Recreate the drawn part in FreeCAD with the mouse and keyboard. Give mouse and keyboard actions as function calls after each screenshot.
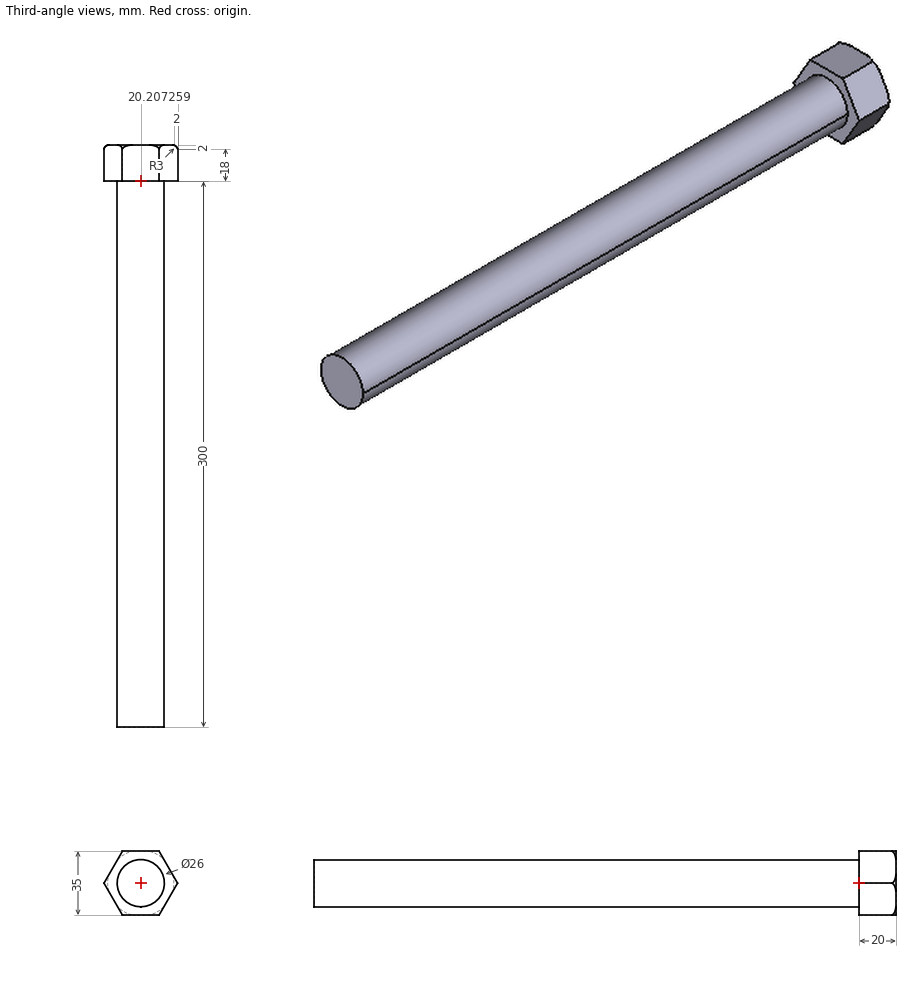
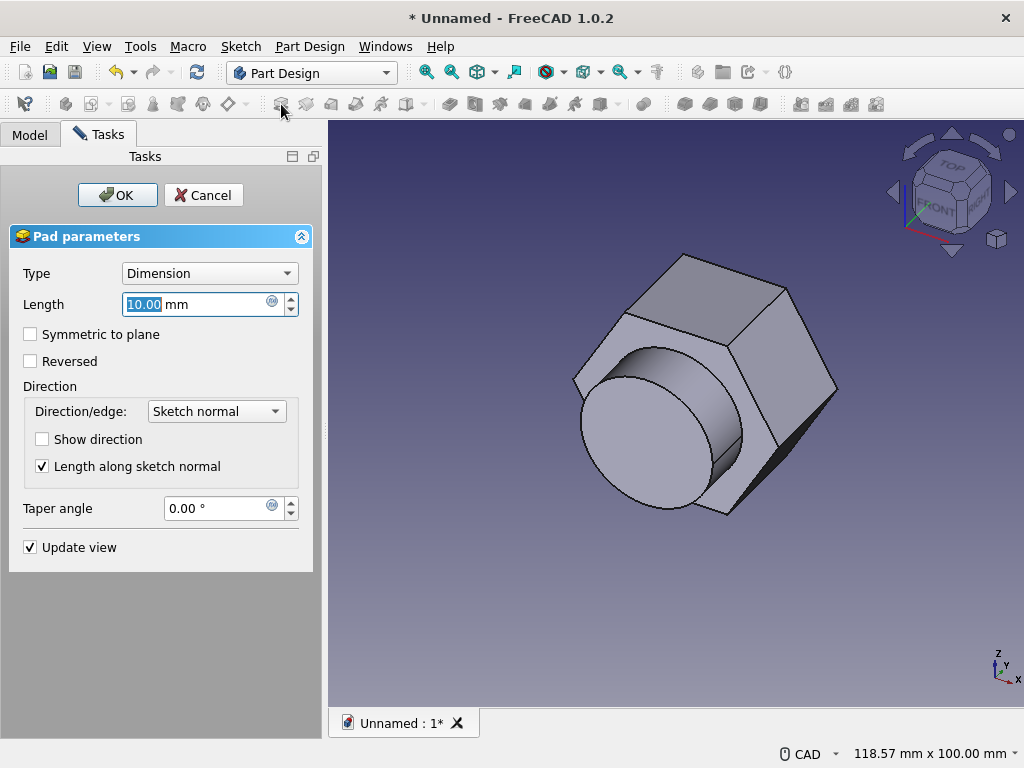
text(300)
key(Tab)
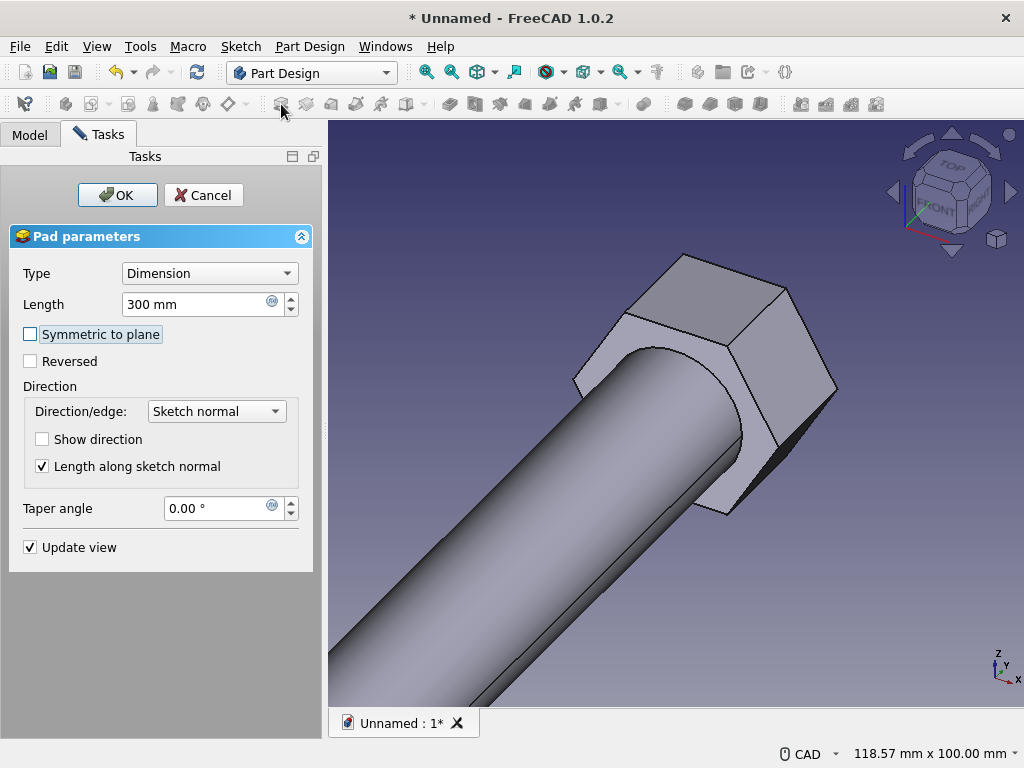
click(118, 195)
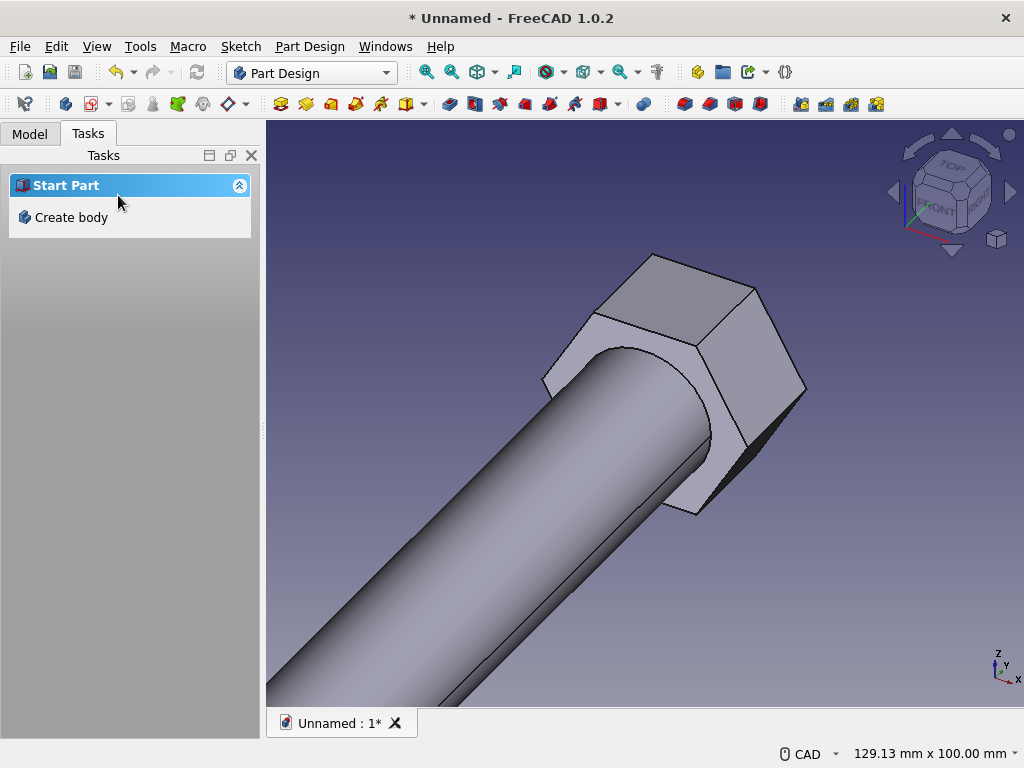
click(427, 72)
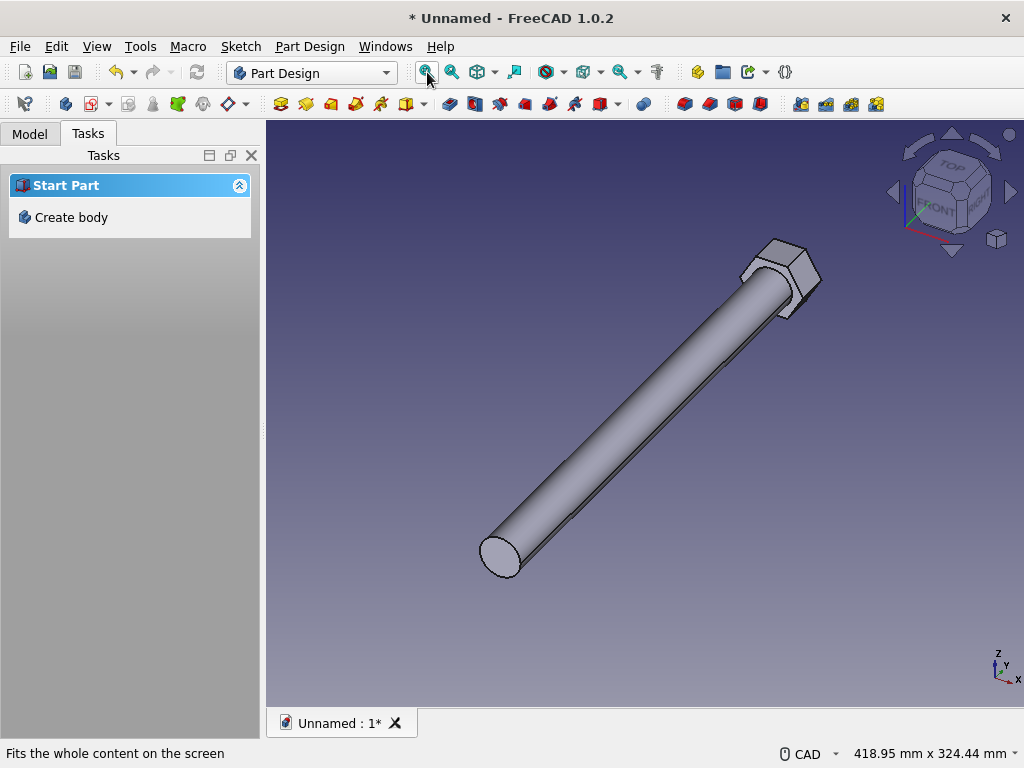
click(90, 104)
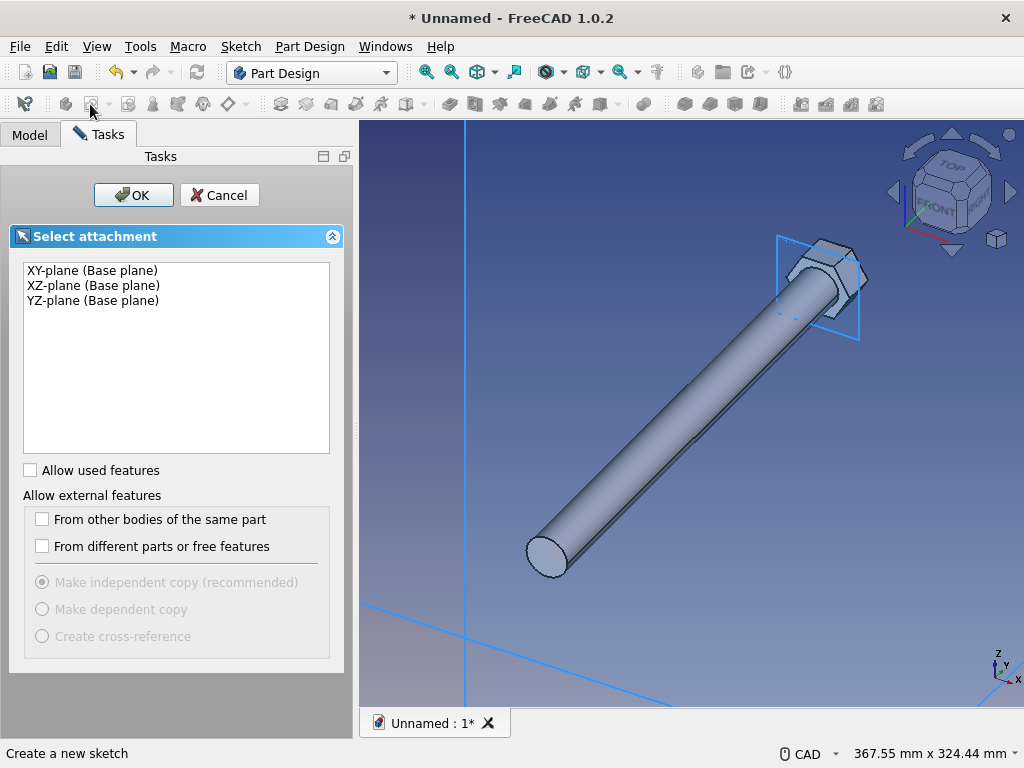
click(84, 270)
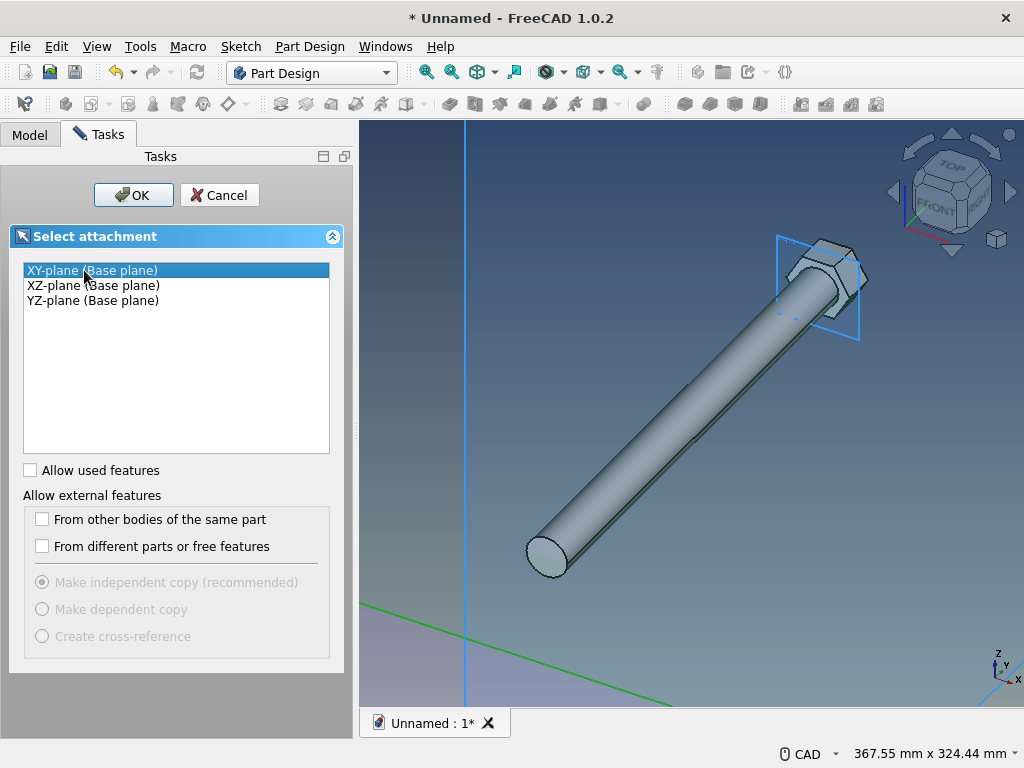
click(134, 195)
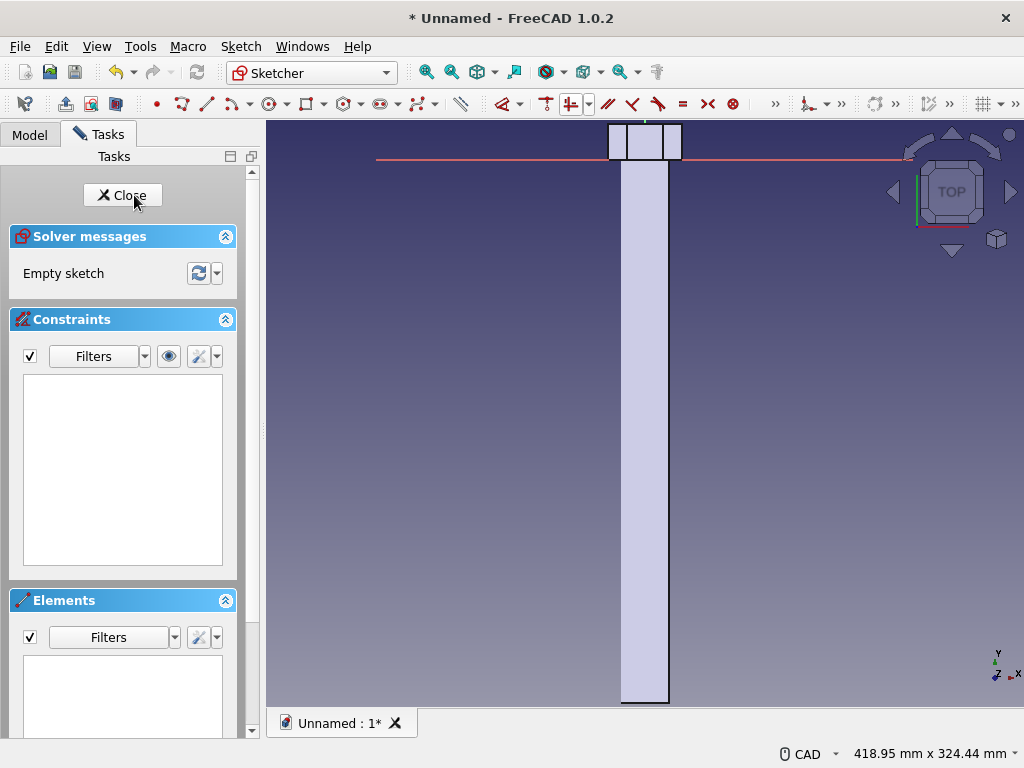
click(116, 104)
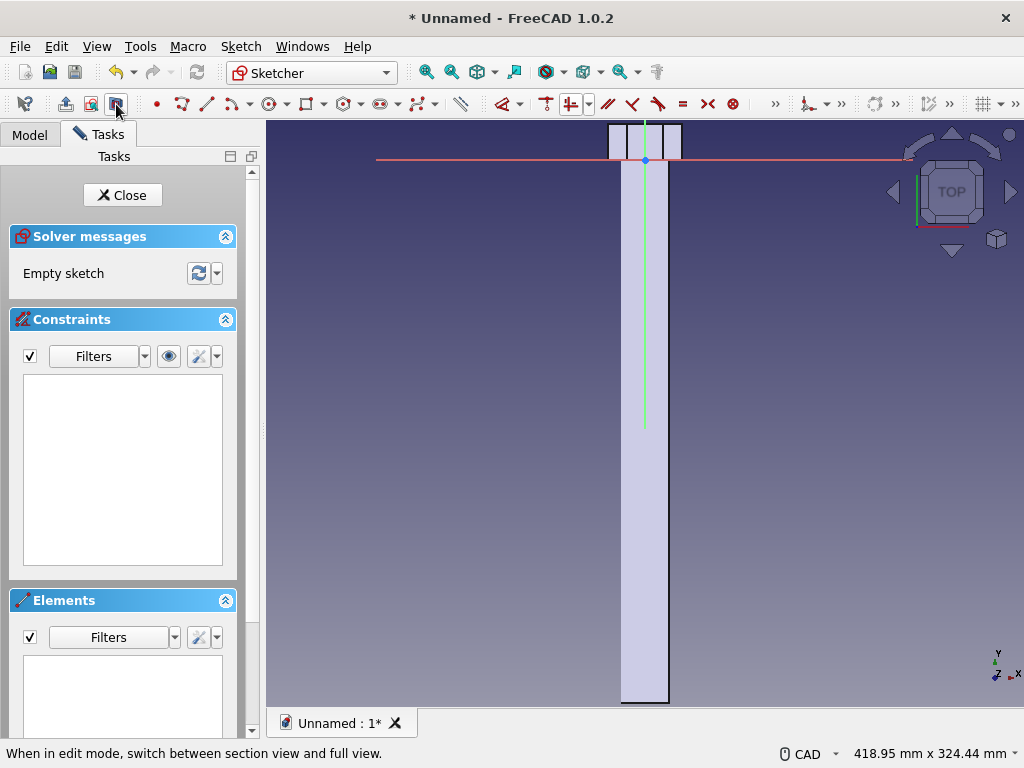
scroll(576, 414, down, 5)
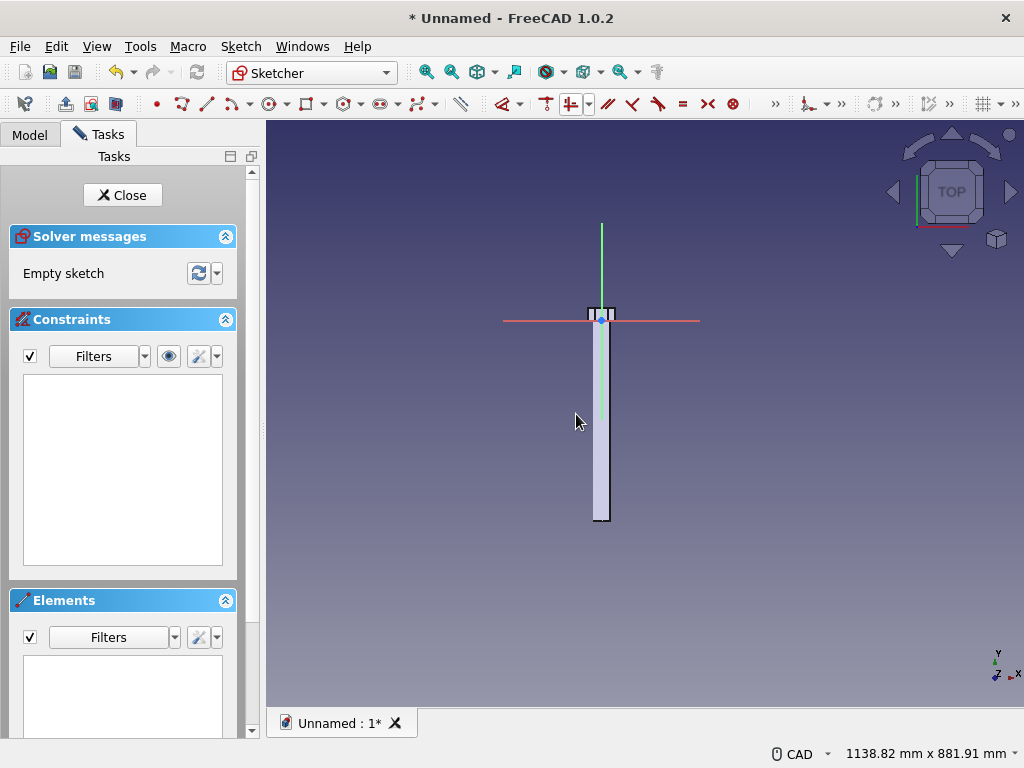
scroll(616, 303, up, 15)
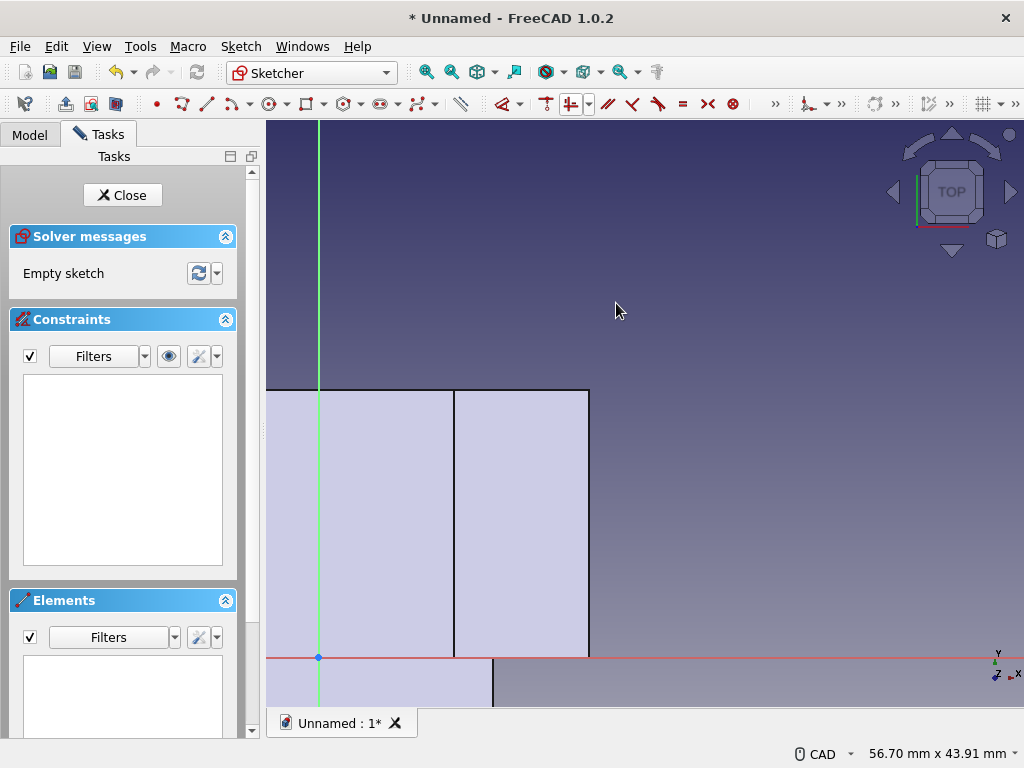
scroll(576, 403, up, 13)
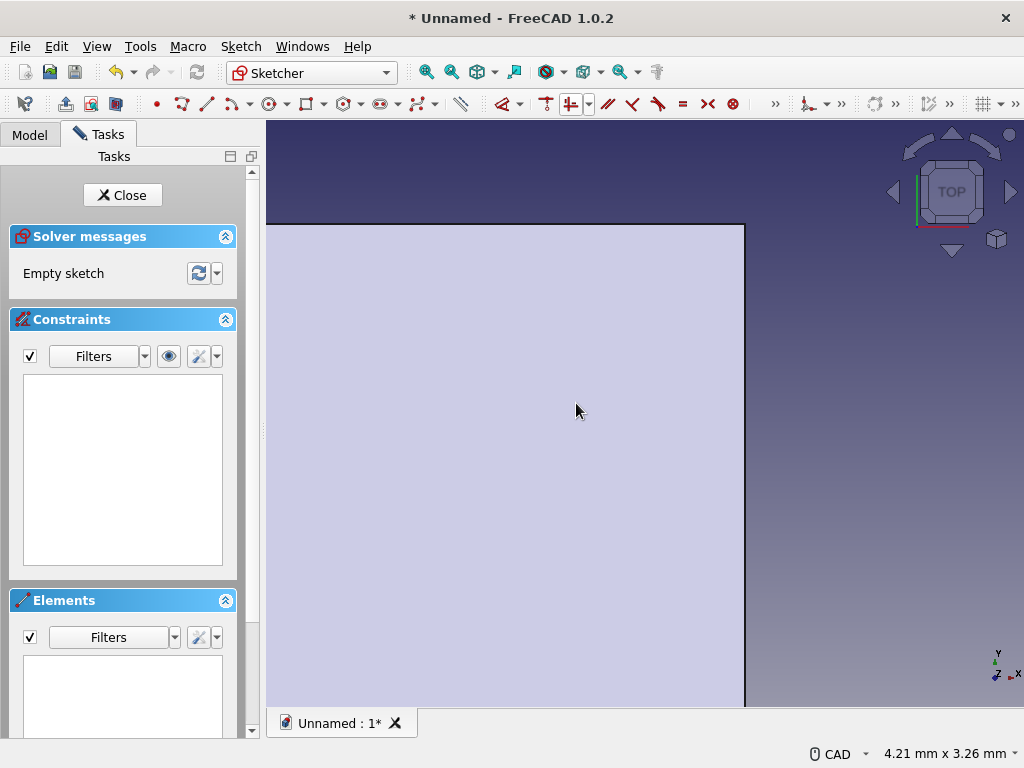
click(182, 104)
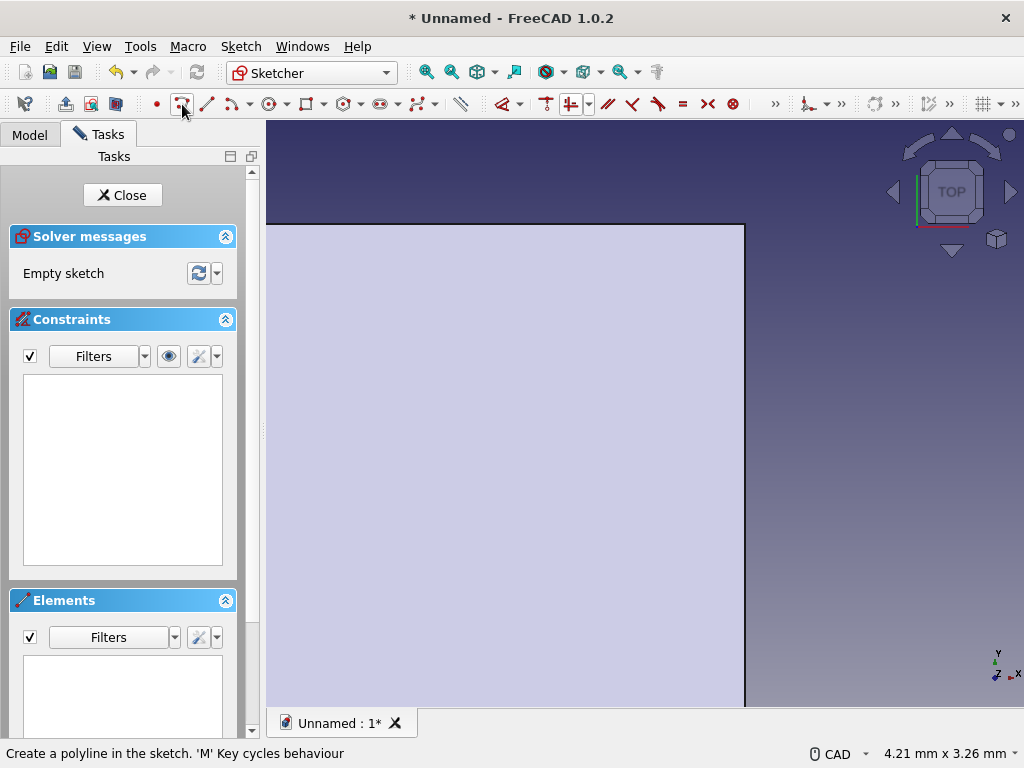
click(745, 584)
click(745, 224)
click(385, 224)
right_click(385, 224)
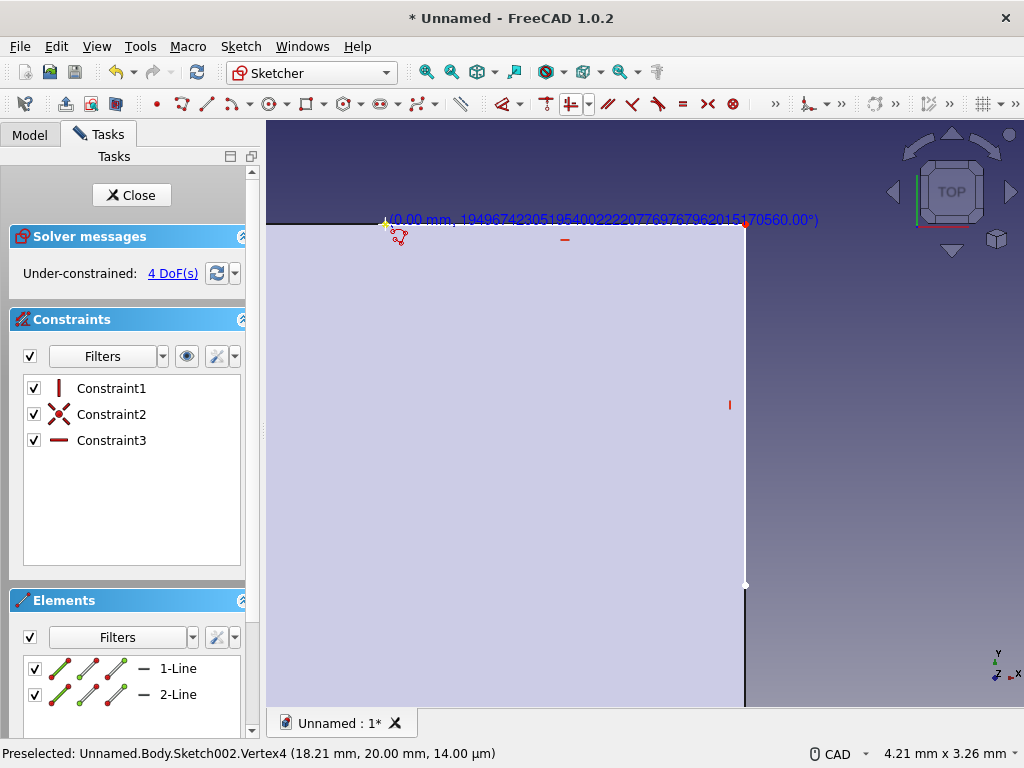
click(250, 104)